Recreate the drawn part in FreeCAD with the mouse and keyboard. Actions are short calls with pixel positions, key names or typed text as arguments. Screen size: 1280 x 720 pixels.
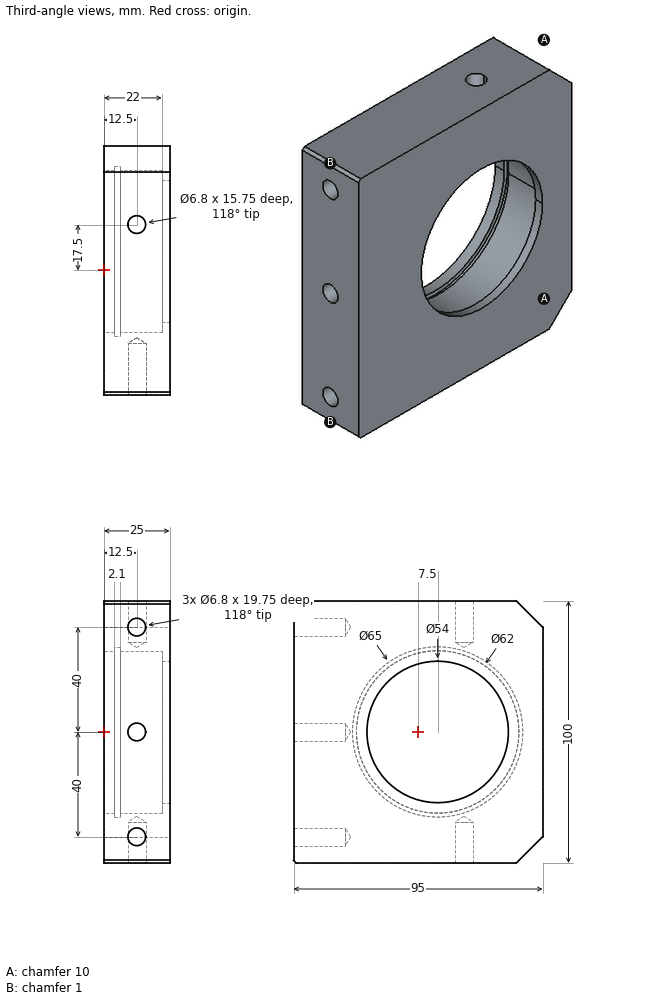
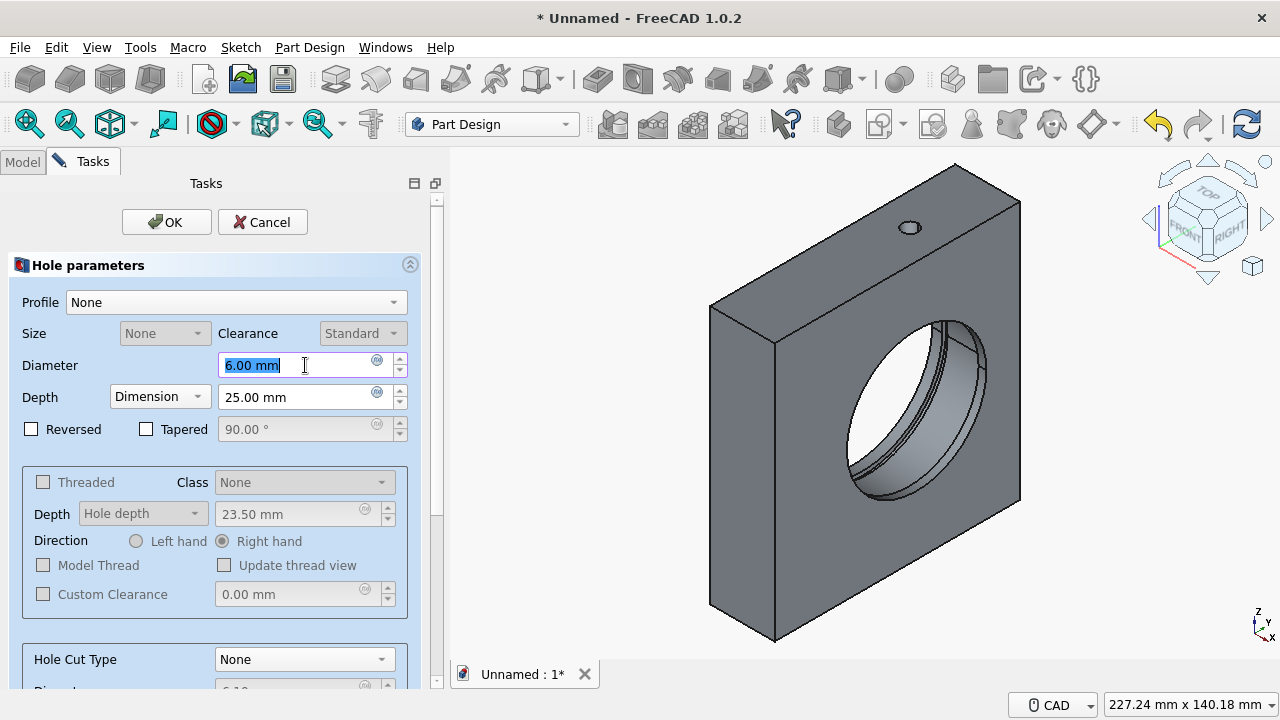
text(6.8)
key(Tab)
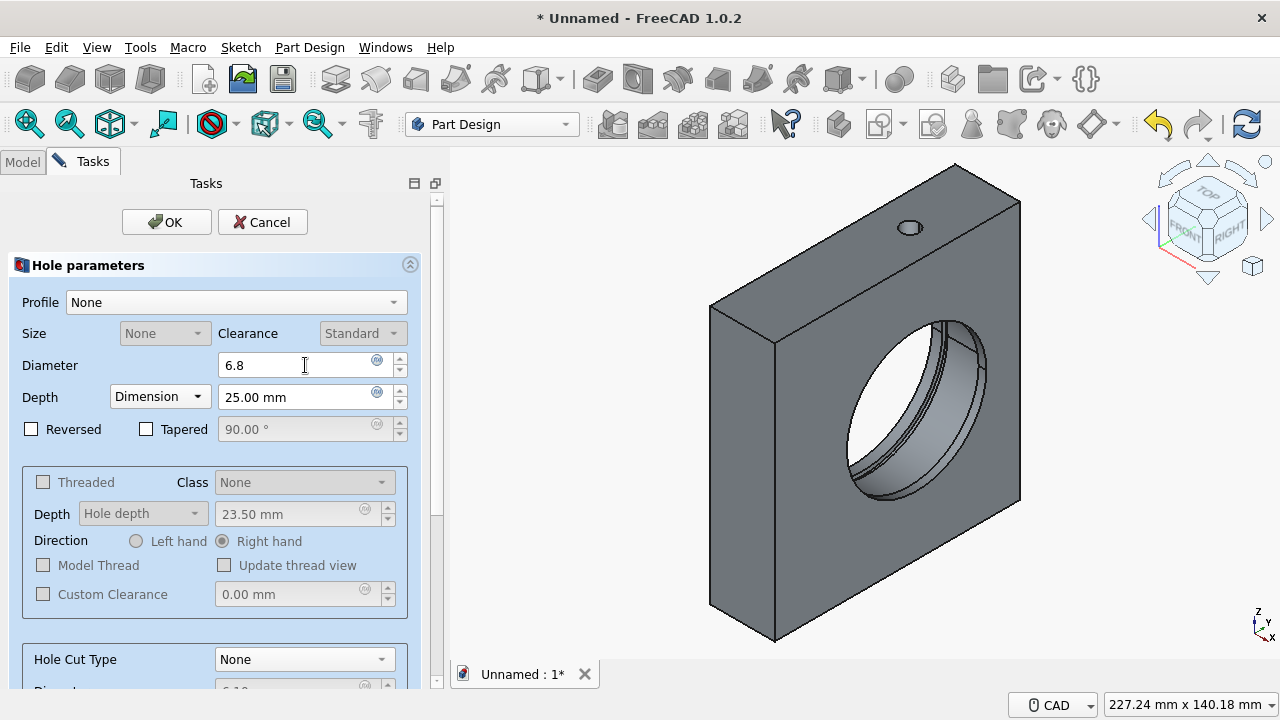
triple_click(305, 397)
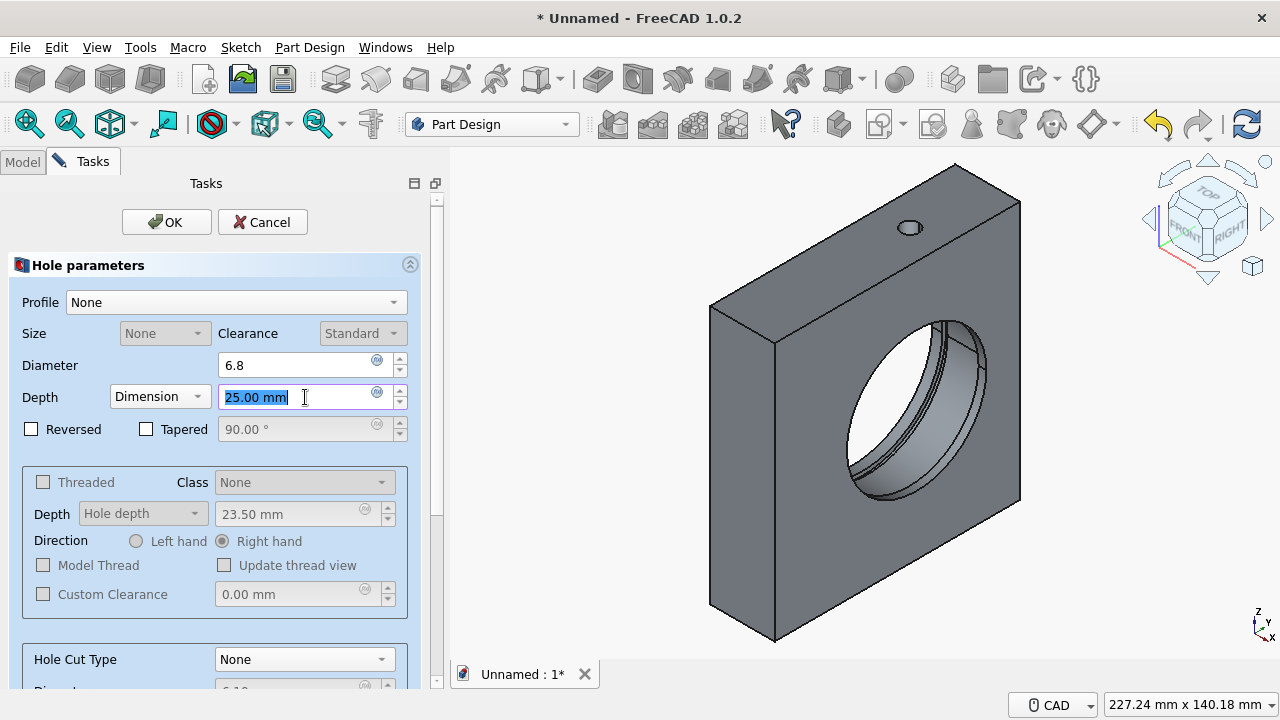
text(15.75)
key(Tab)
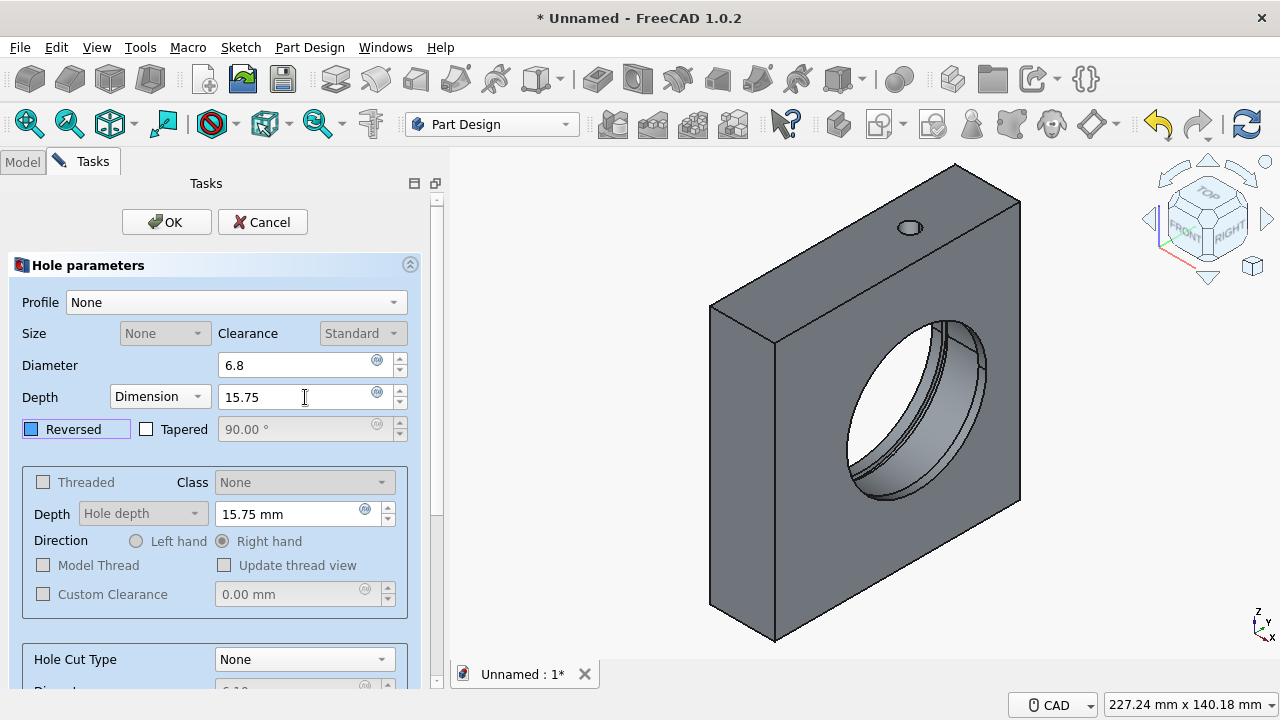
click(167, 222)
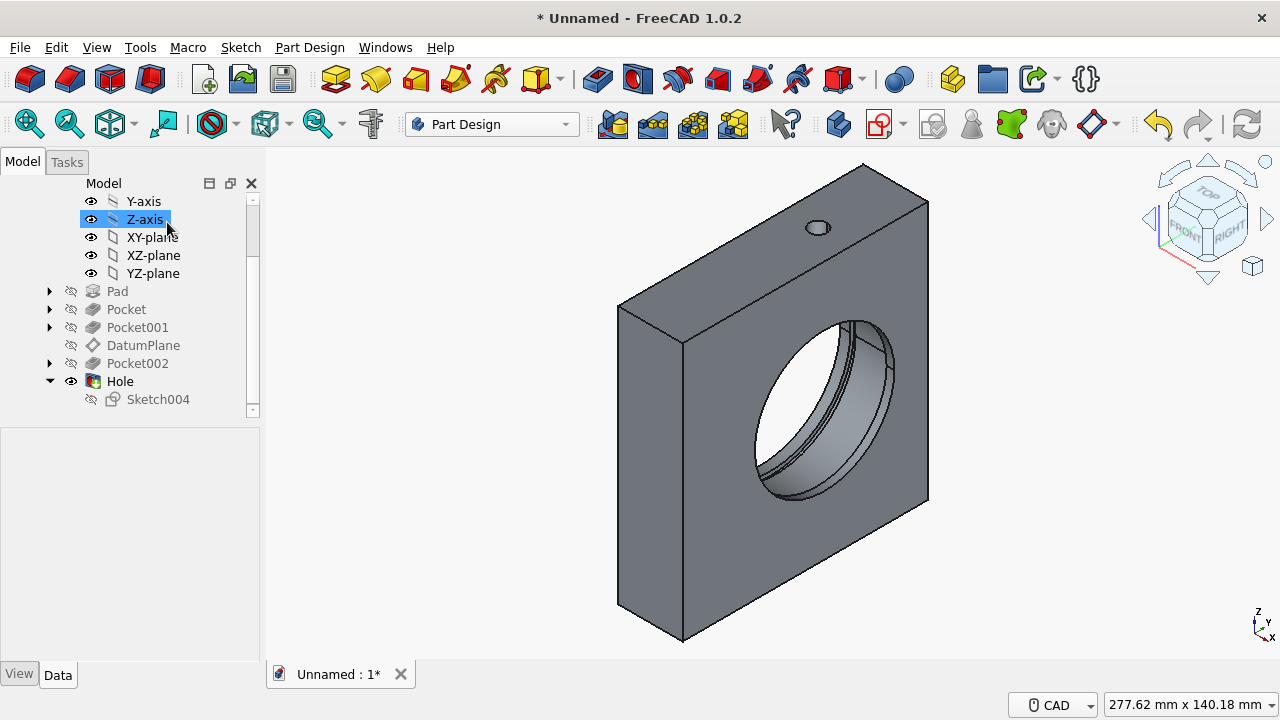
key(5)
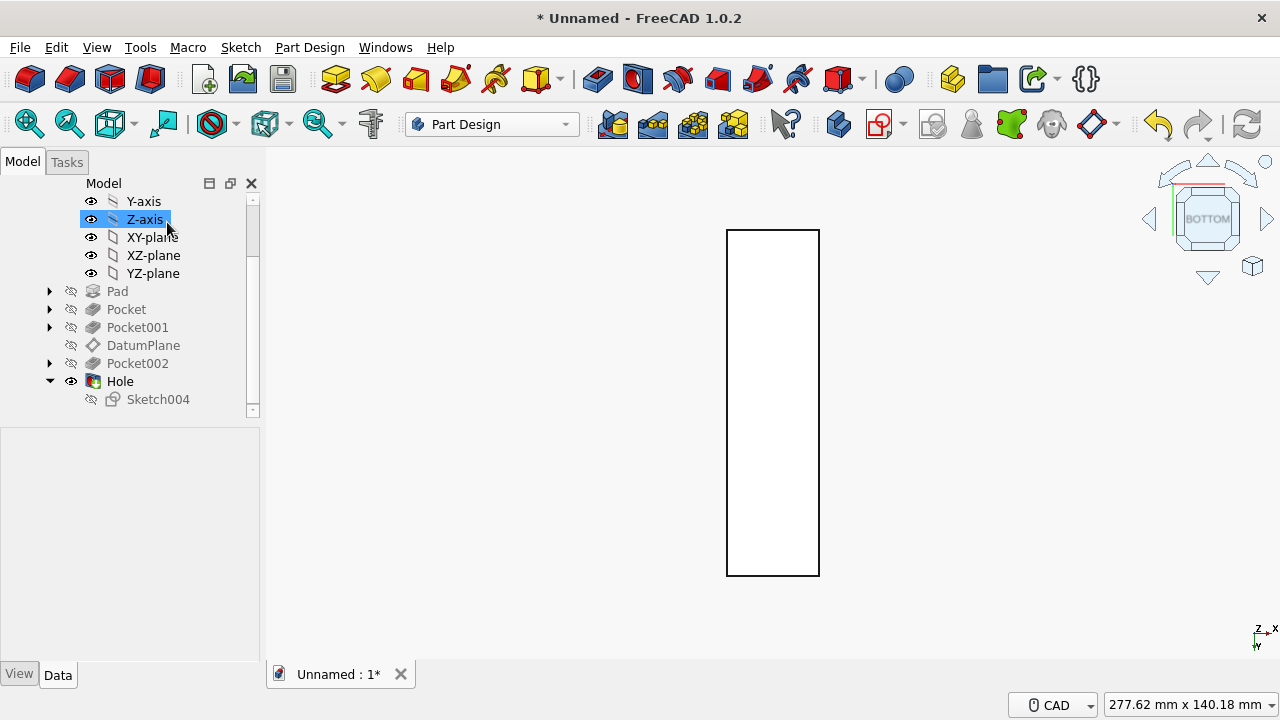
click(773, 501)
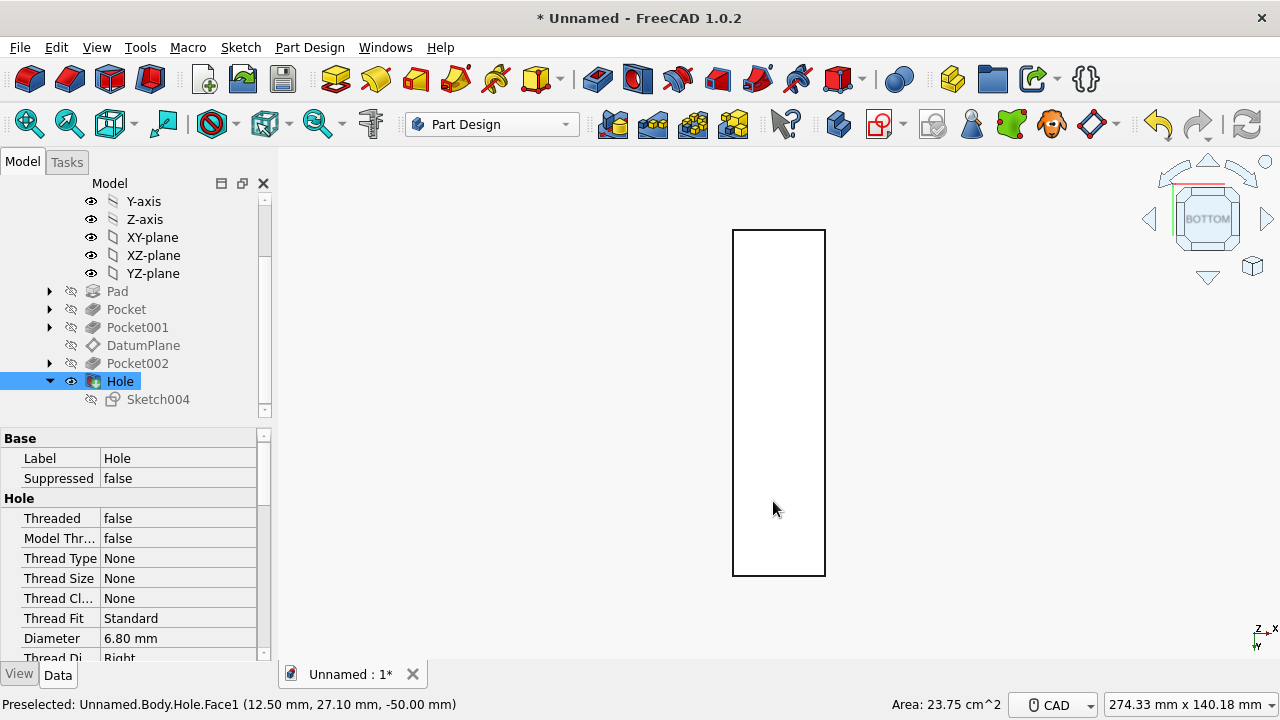
click(880, 124)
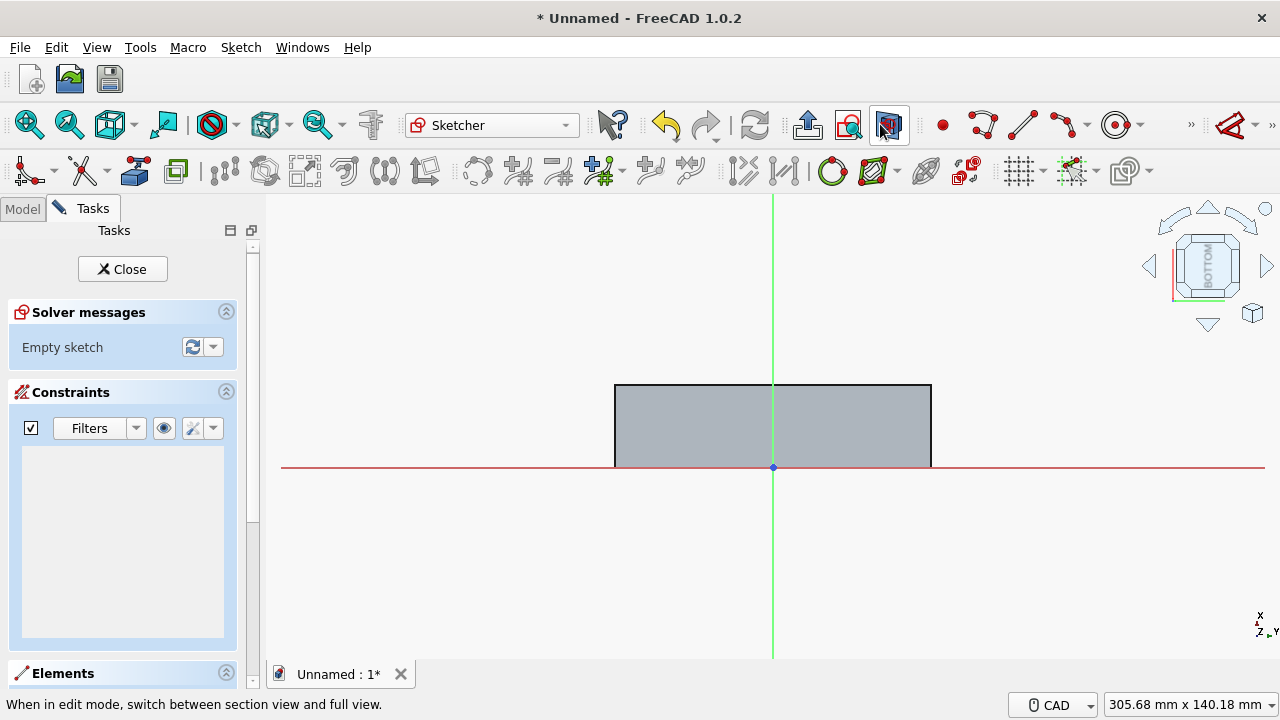
scroll(841, 427, up, 13)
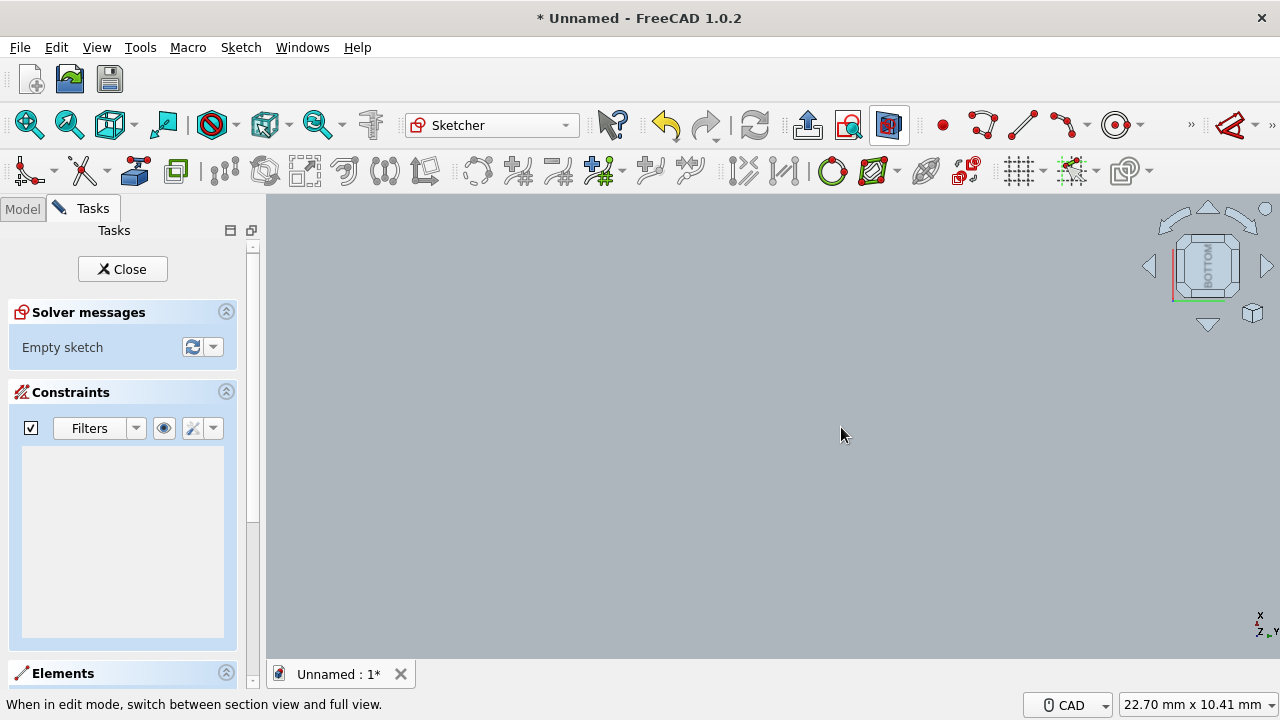
click(1116, 126)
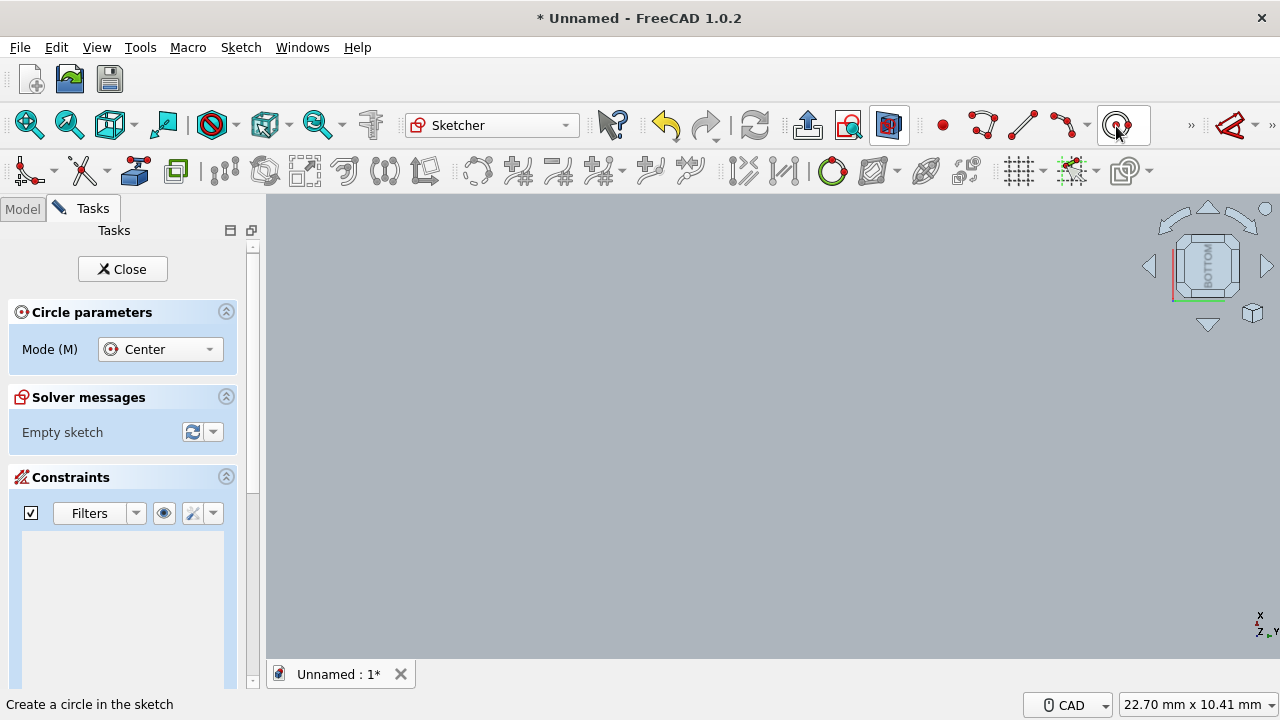
click(700, 414)
click(807, 307)
key(Escape)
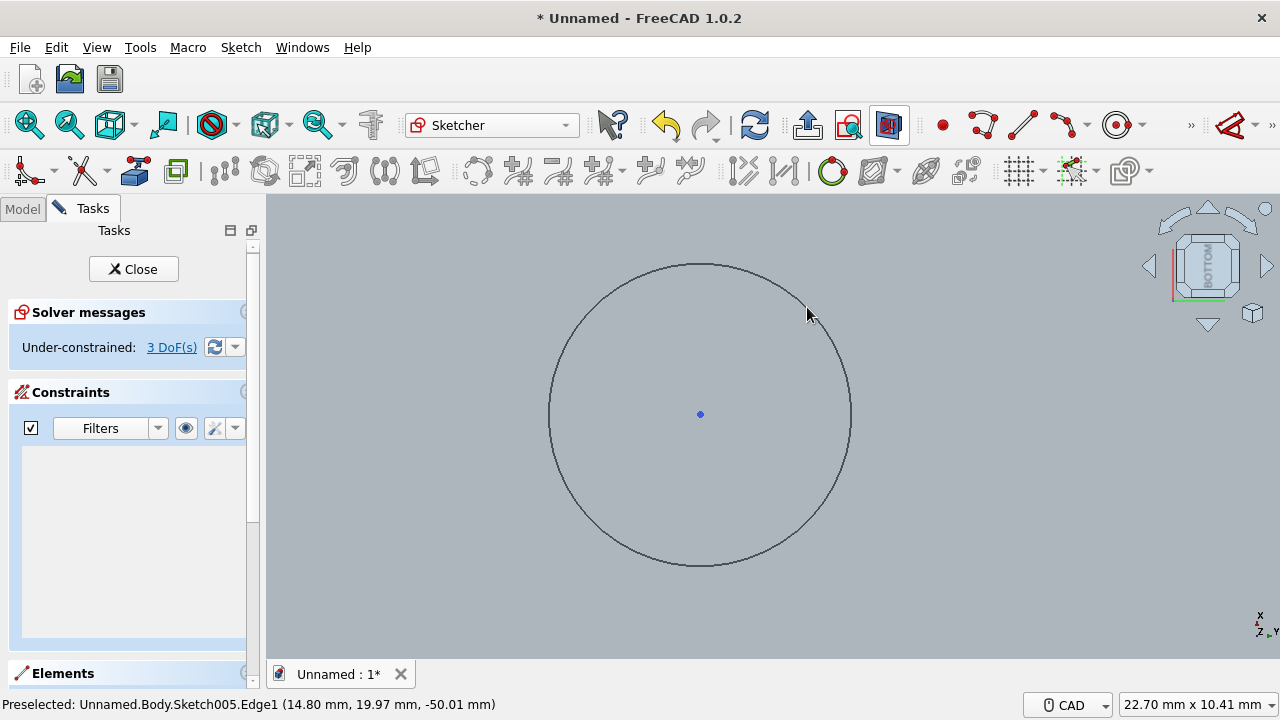
click(1230, 126)